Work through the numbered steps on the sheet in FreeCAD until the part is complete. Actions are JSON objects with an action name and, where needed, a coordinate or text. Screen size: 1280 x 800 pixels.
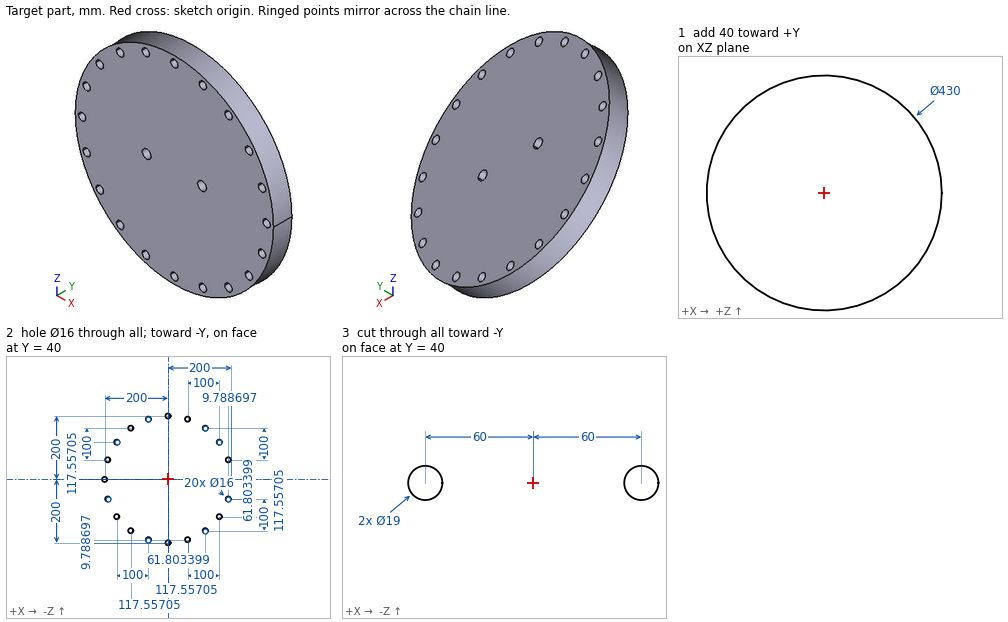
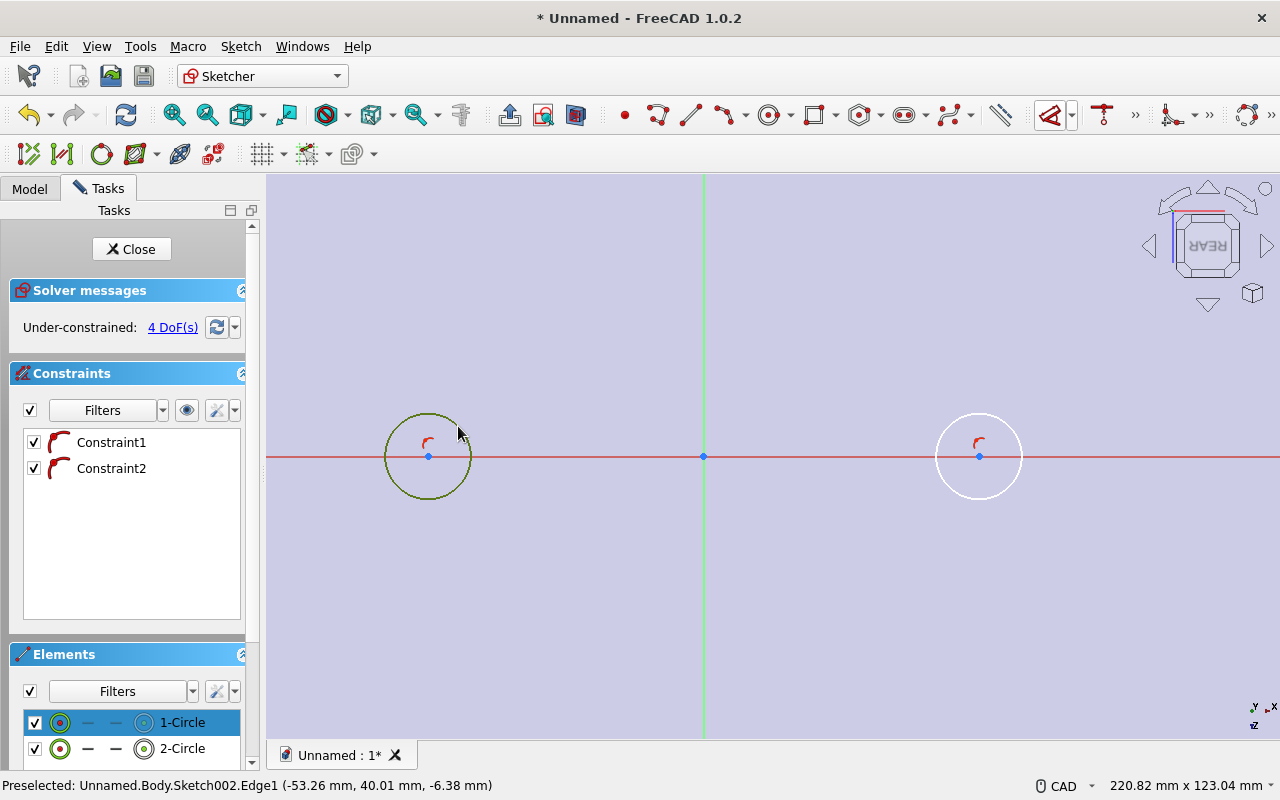
{"action": "left_click", "coordinate": [1009, 426]}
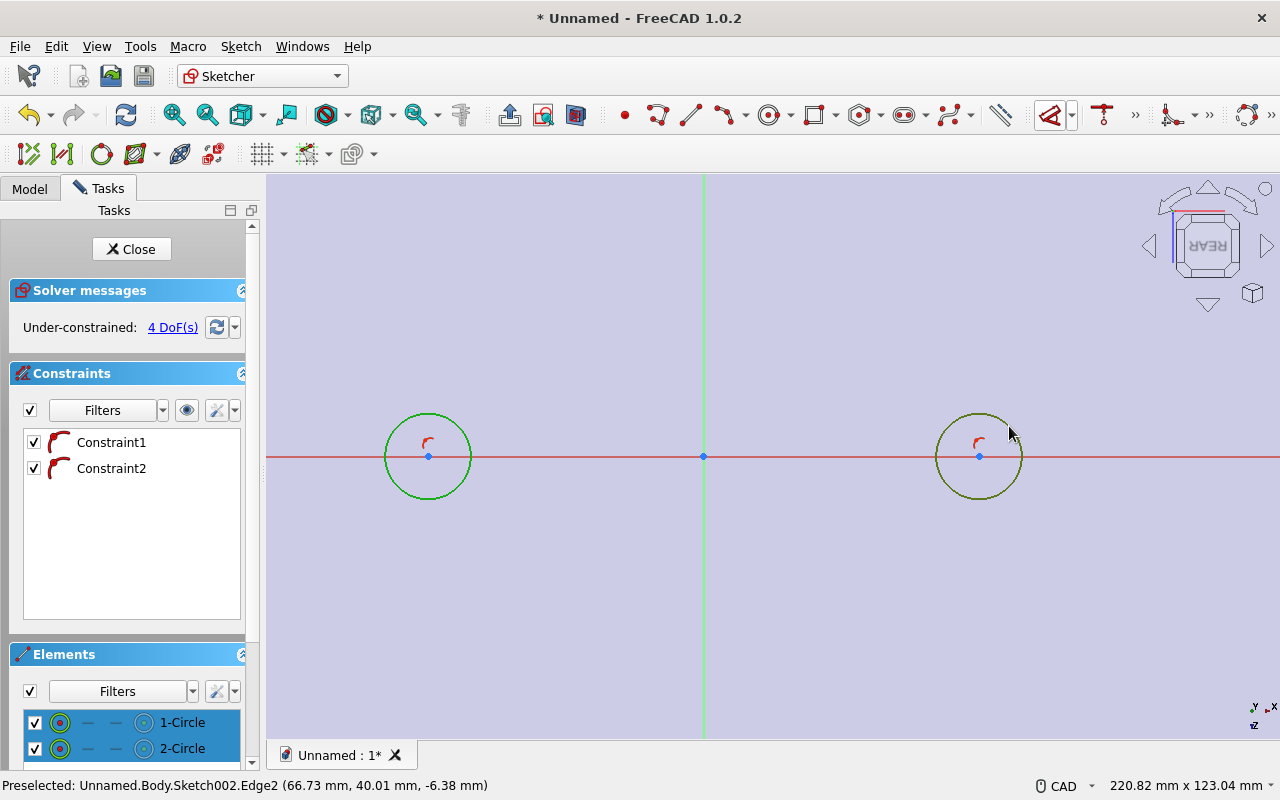
{"action": "key", "text": "e"}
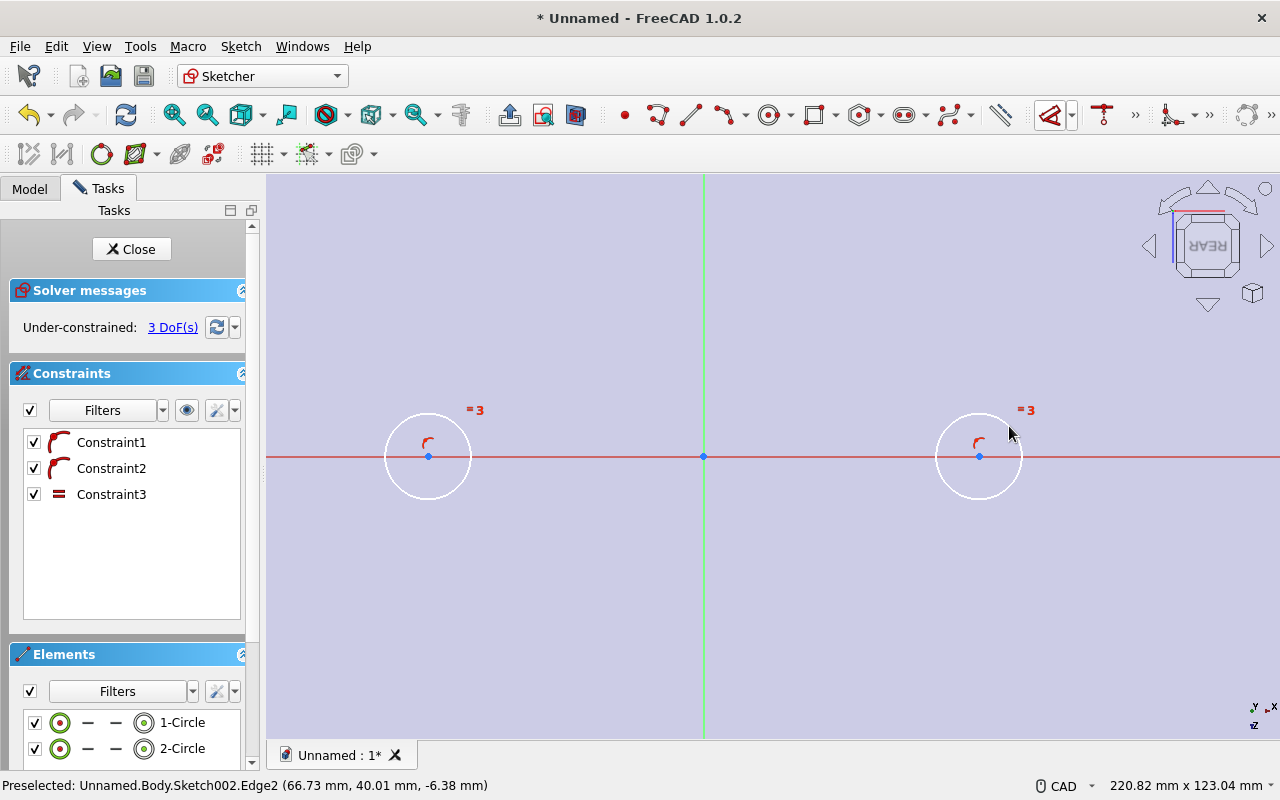
{"action": "key", "text": "d"}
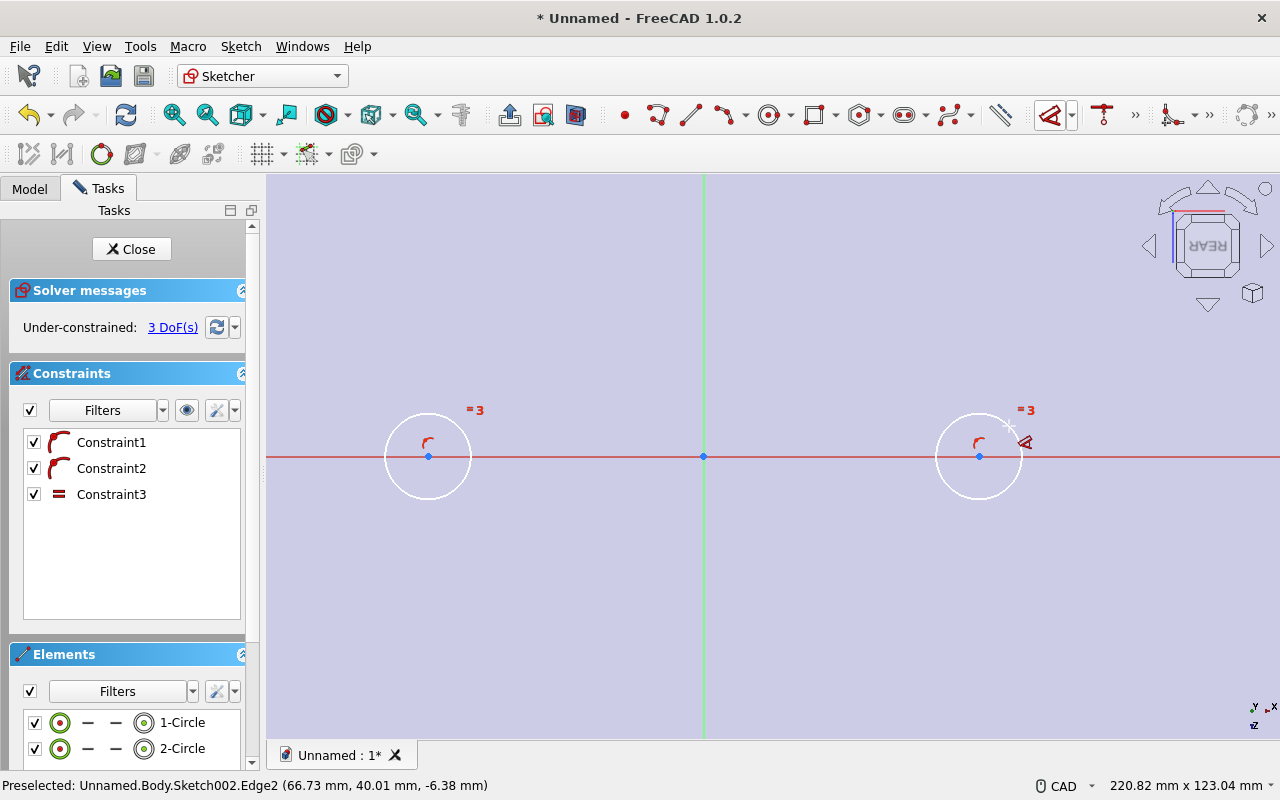
{"action": "left_click", "coordinate": [458, 426]}
{"action": "left_click", "coordinate": [480, 403]}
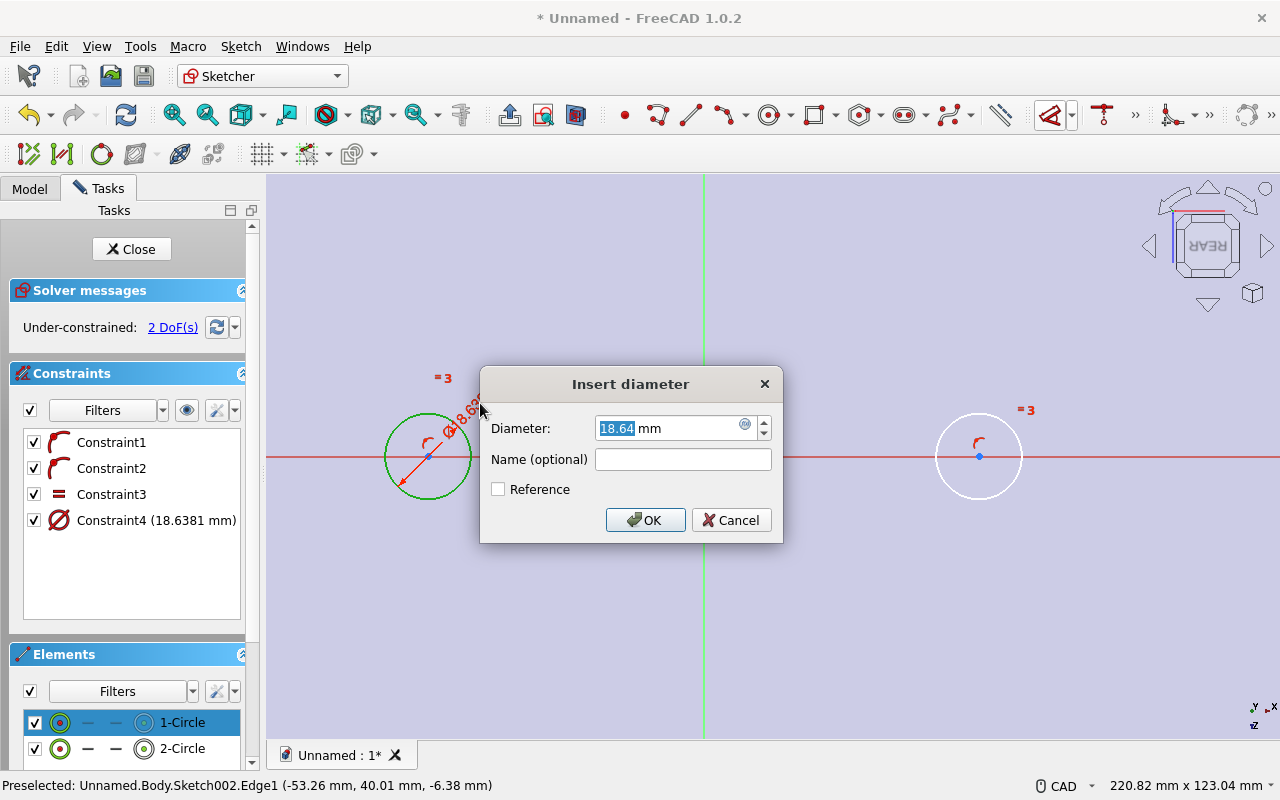
{"action": "type", "text": "19"}
{"action": "key", "text": "Return"}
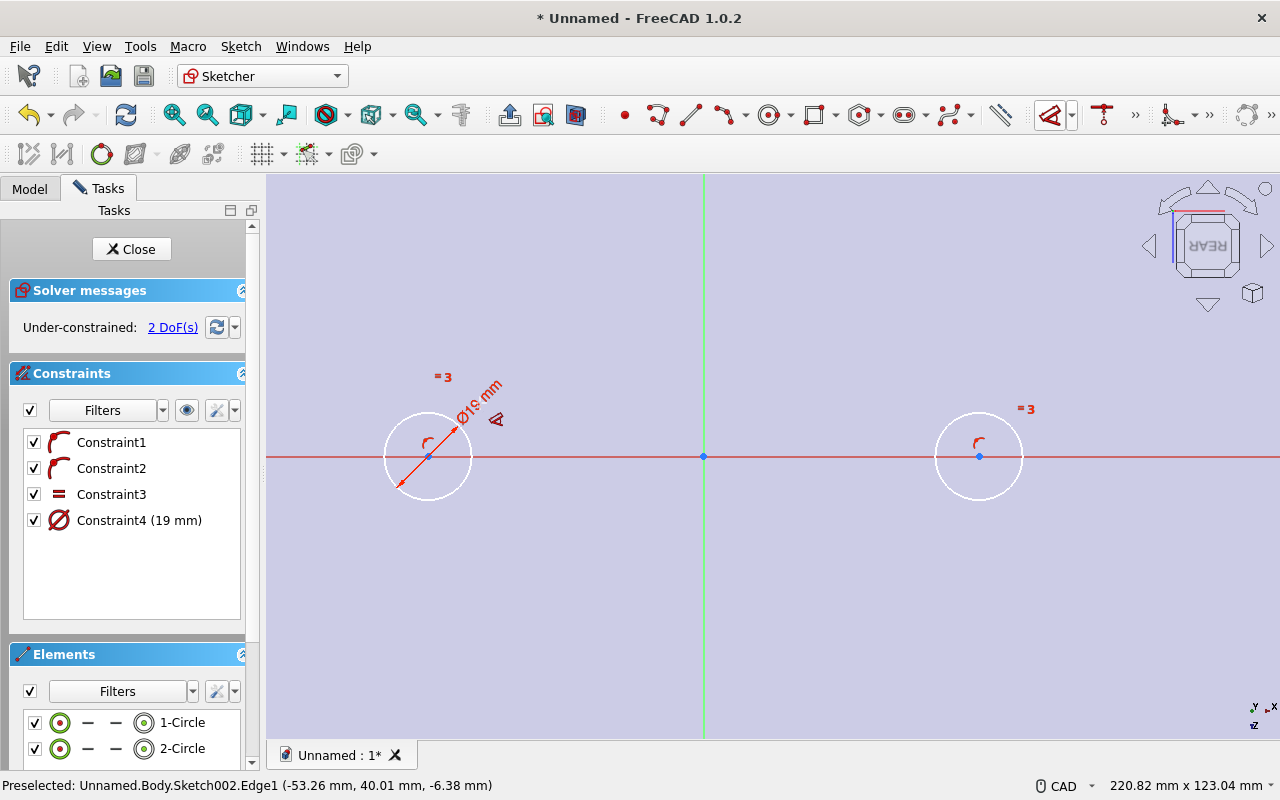
{"action": "left_click", "coordinate": [428, 456]}
{"action": "left_click", "coordinate": [566, 490]}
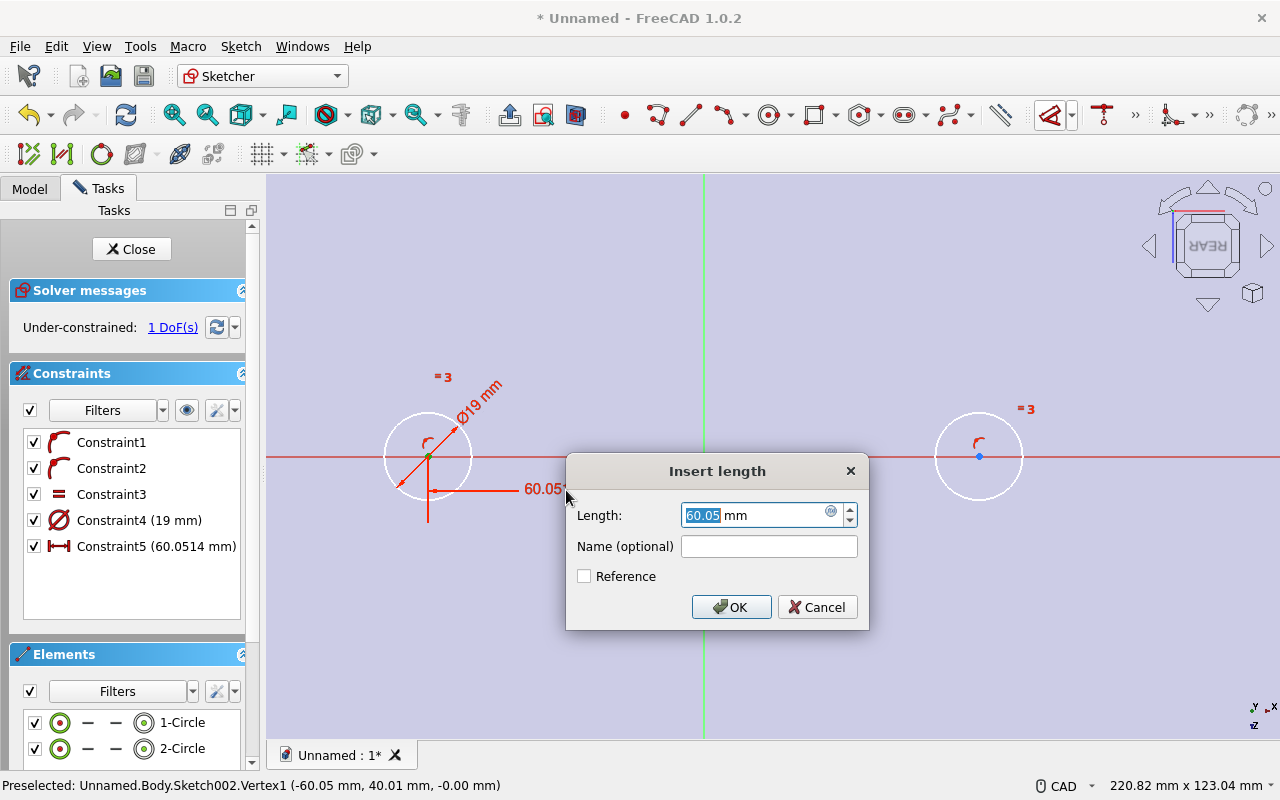
{"action": "type", "text": "60"}
{"action": "key", "text": "Return"}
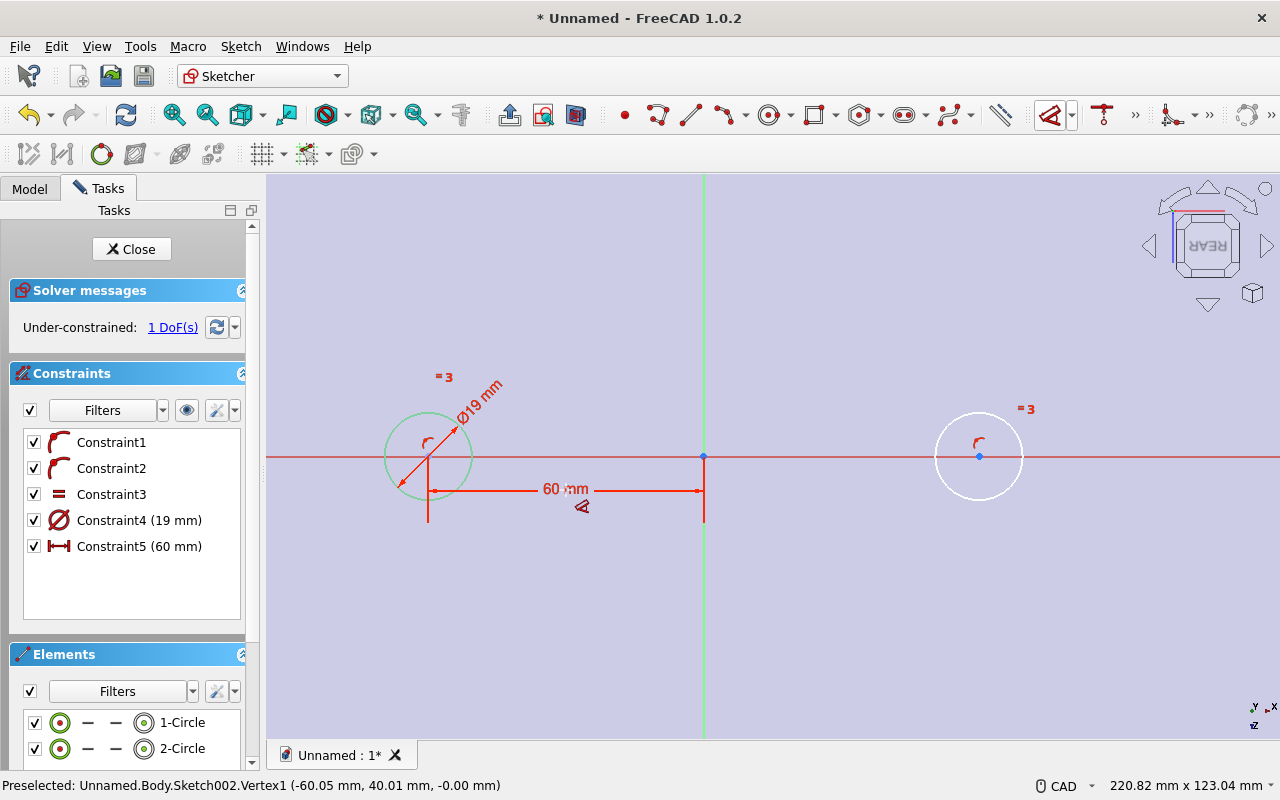
{"action": "left_click", "coordinate": [979, 456]}
{"action": "left_click", "coordinate": [841, 490]}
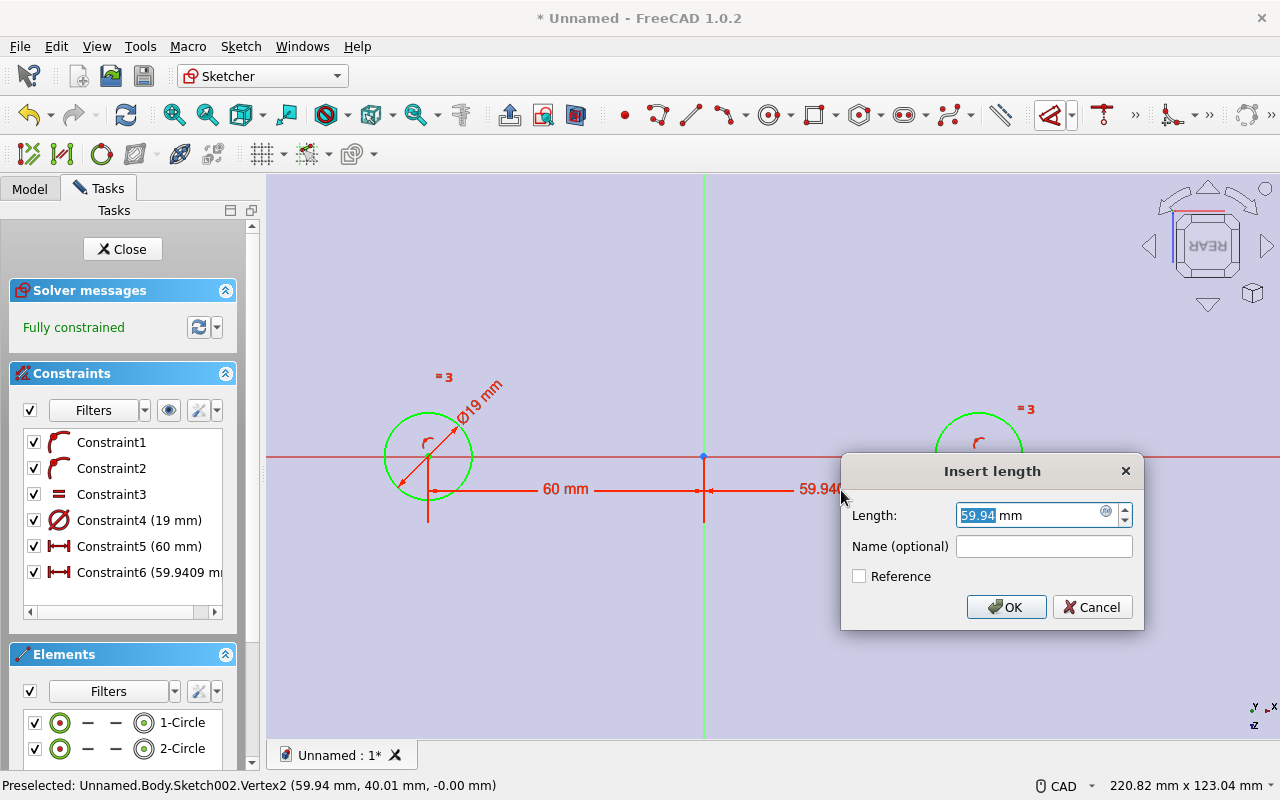
{"action": "type", "text": "60"}
{"action": "key", "text": "Return"}
{"action": "key", "text": "Escape"}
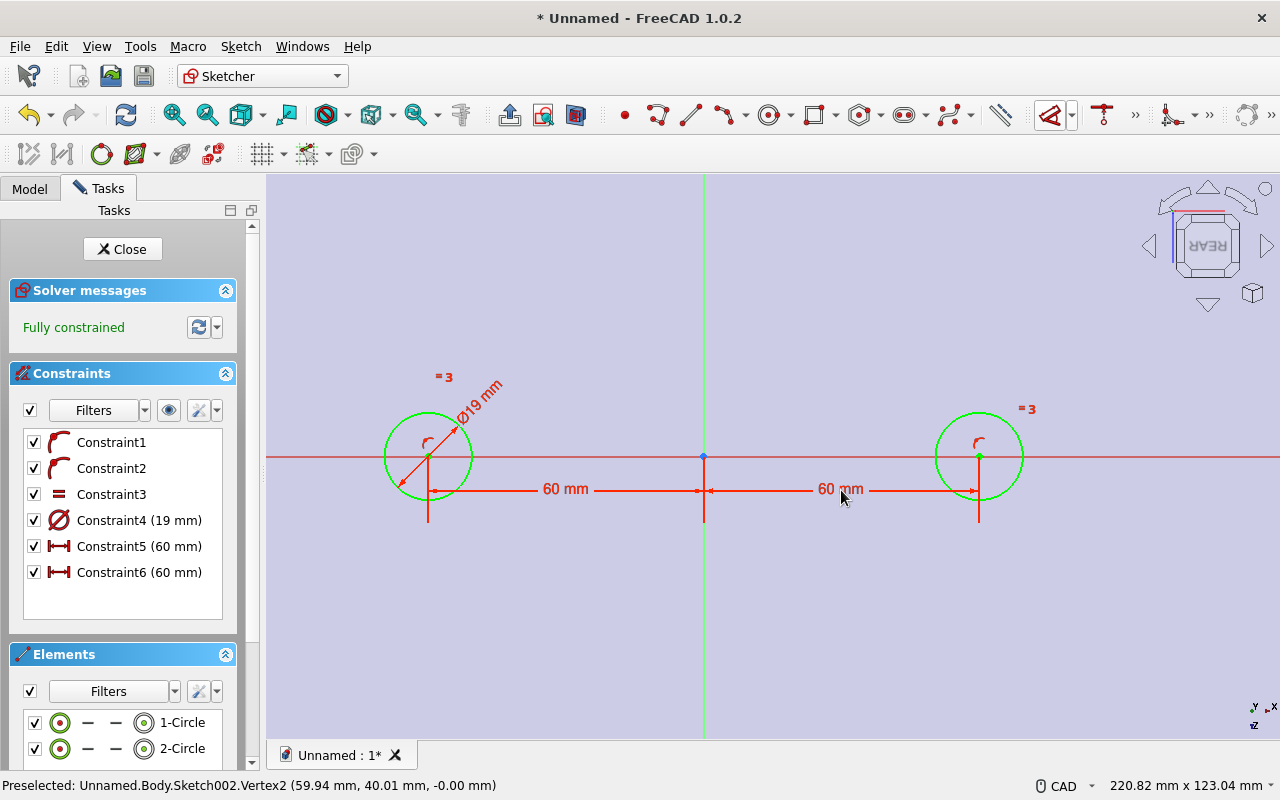
{"action": "left_click", "coordinate": [123, 249]}